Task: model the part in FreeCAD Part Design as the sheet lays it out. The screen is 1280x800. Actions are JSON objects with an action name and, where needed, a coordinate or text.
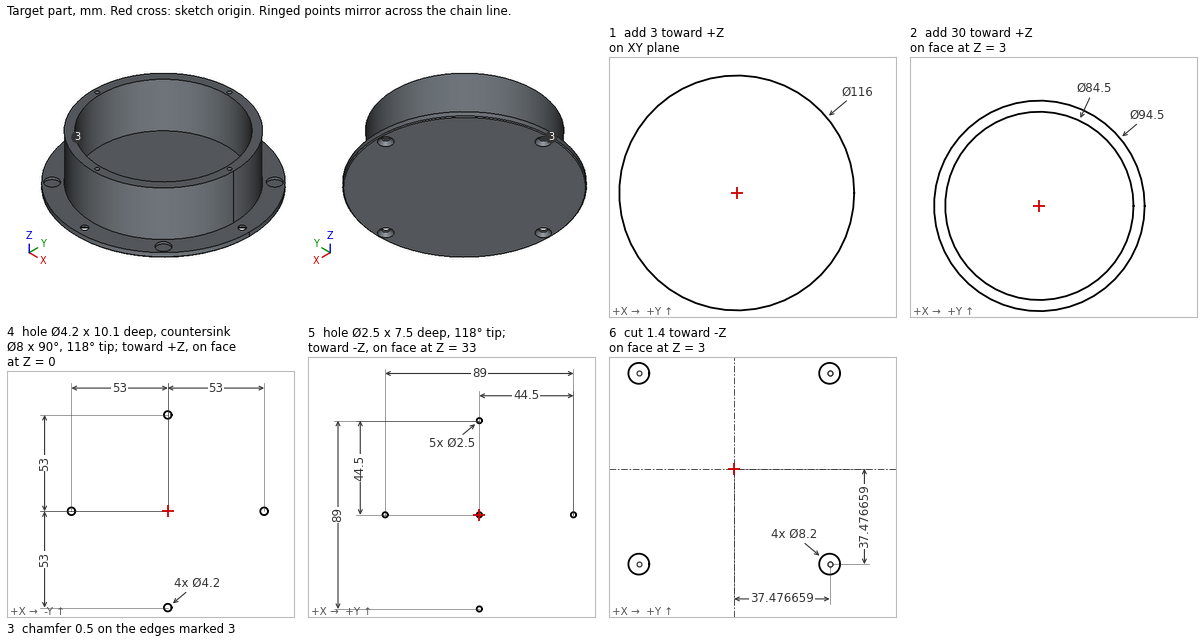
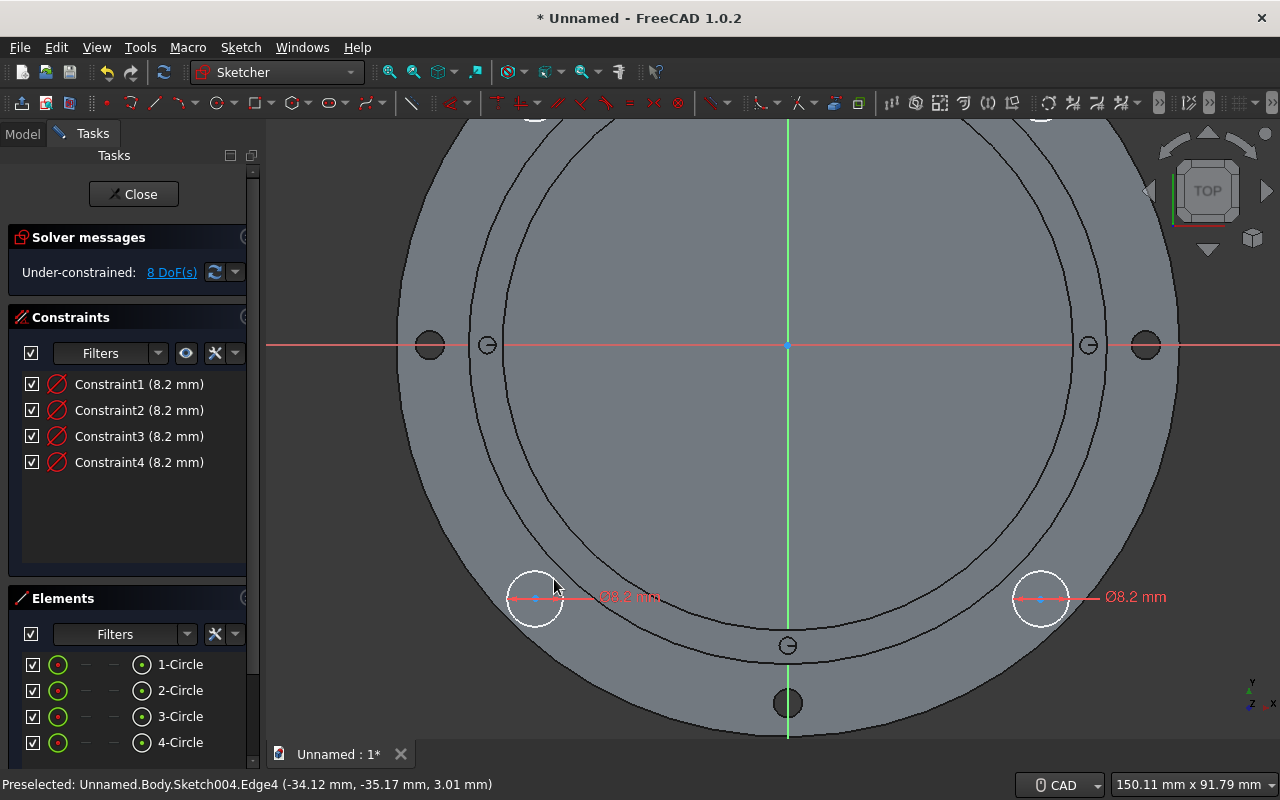
{"action": "left_click", "coordinate": [1041, 599]}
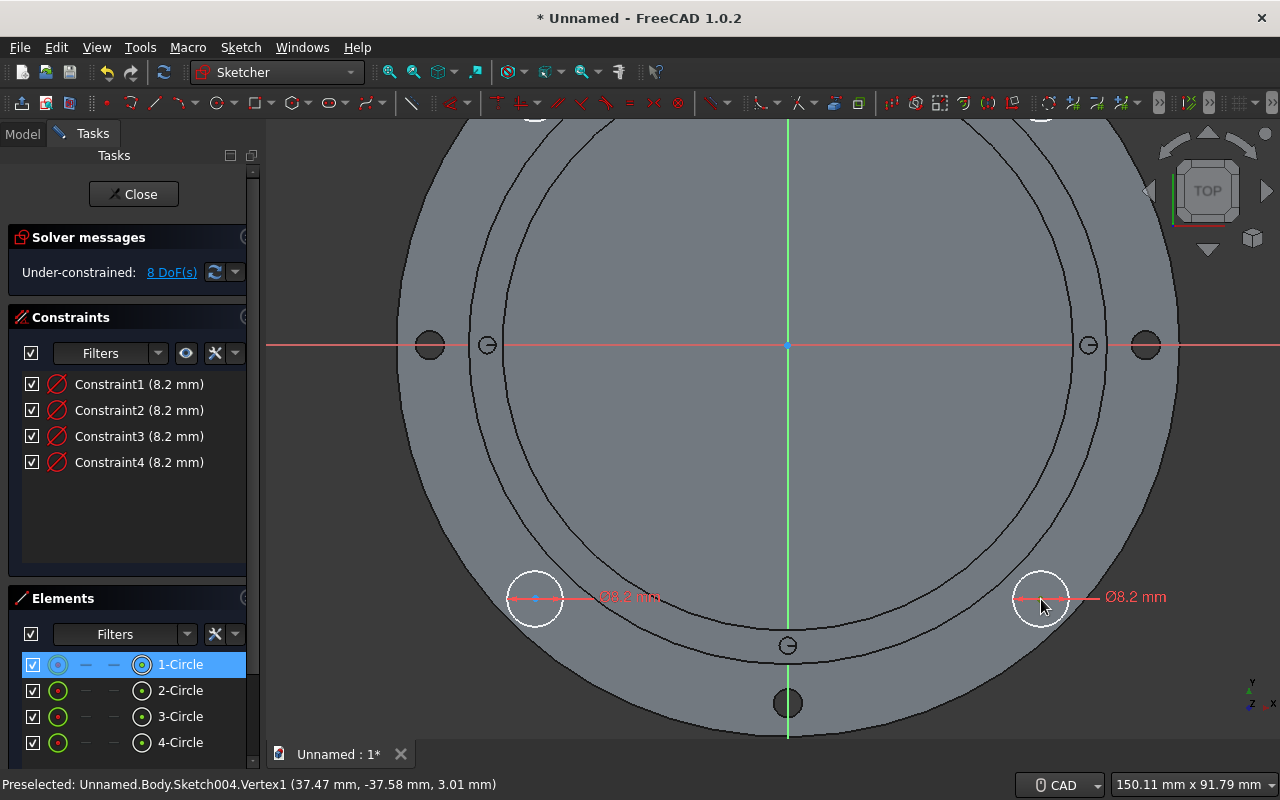
{"action": "scroll", "coordinate": [535, 599], "scroll_direction": "down", "scroll_amount": 2}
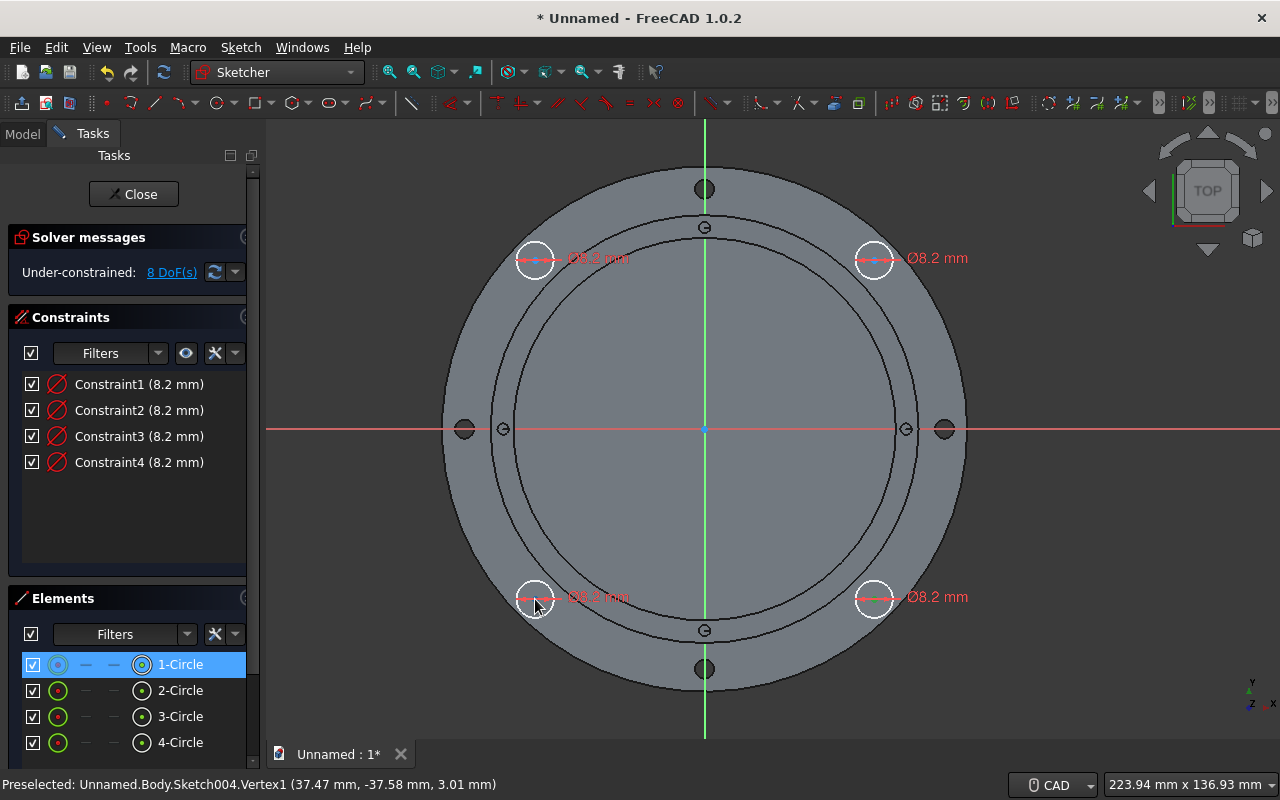
{"action": "left_click", "coordinate": [874, 260]}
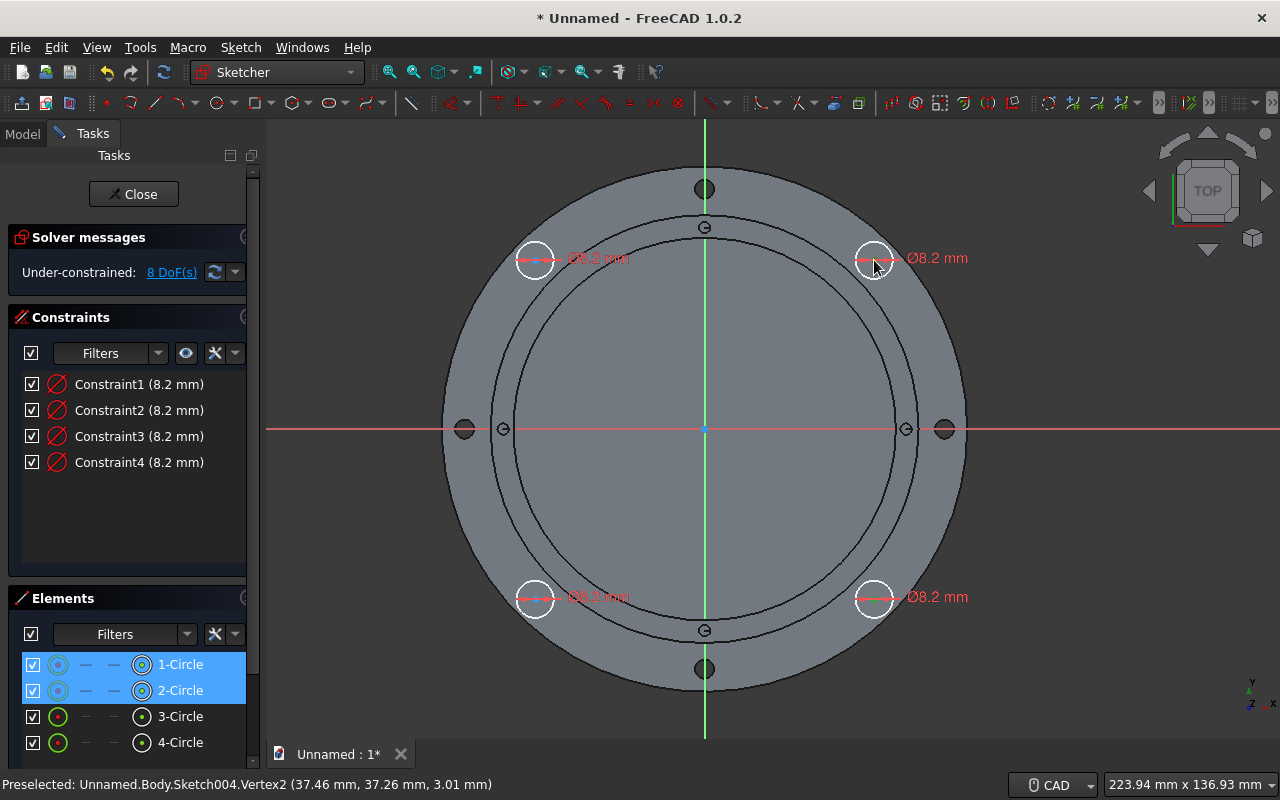
{"action": "left_click", "coordinate": [353, 429]}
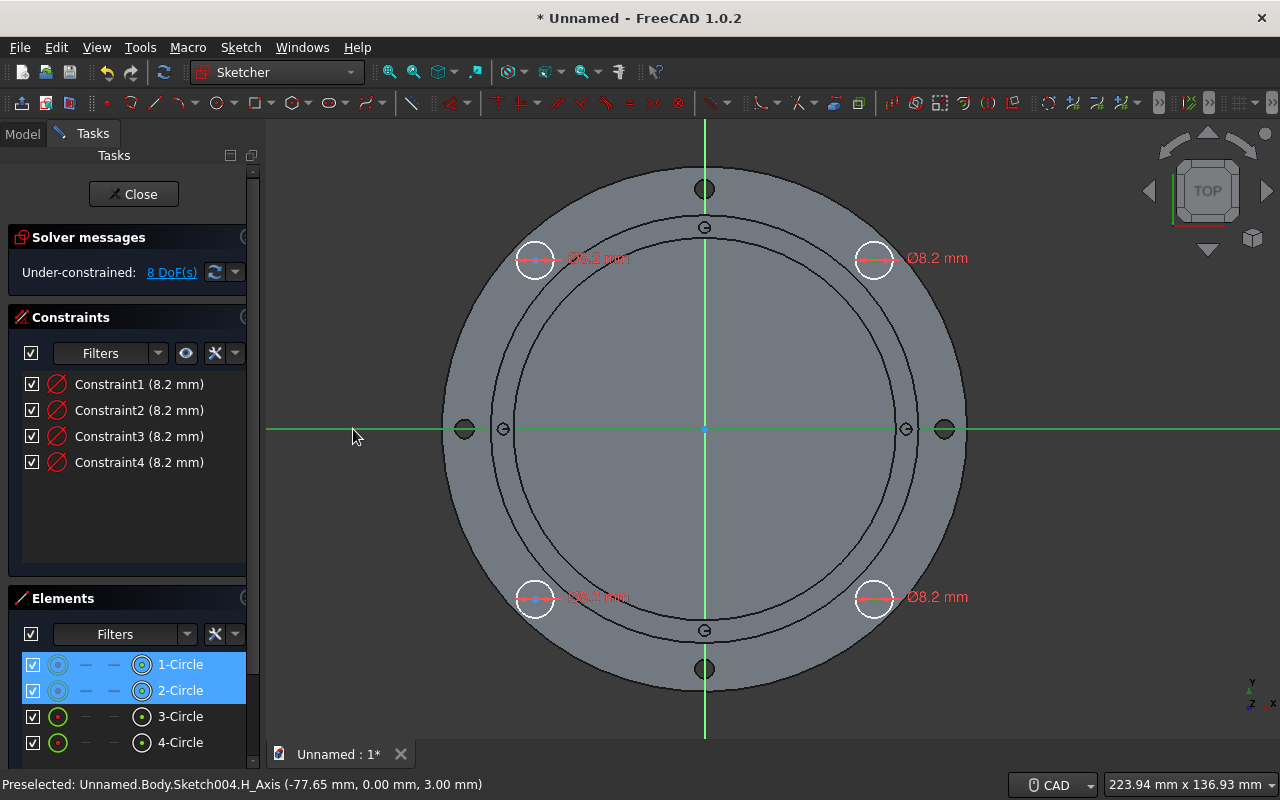
{"action": "left_click", "coordinate": [654, 104]}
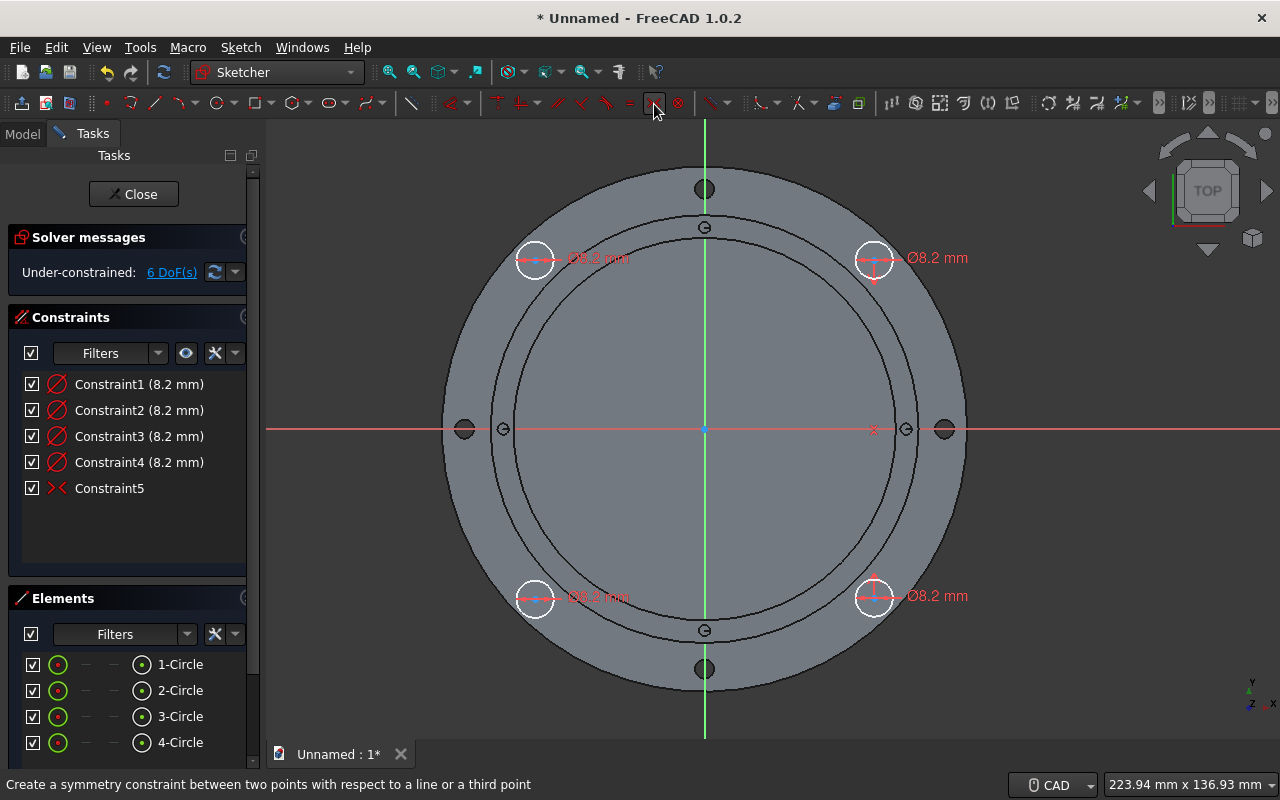
{"action": "left_click", "coordinate": [874, 260]}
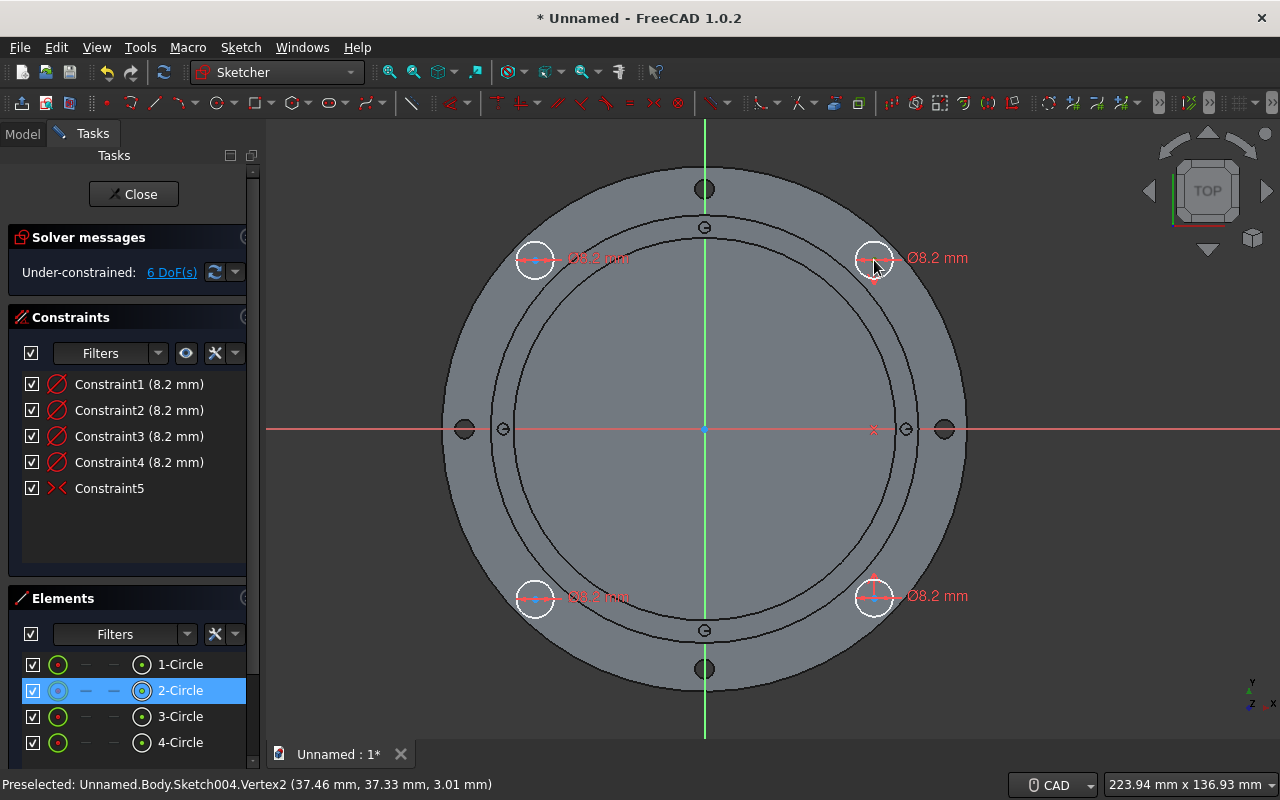
{"action": "left_click", "coordinate": [535, 260]}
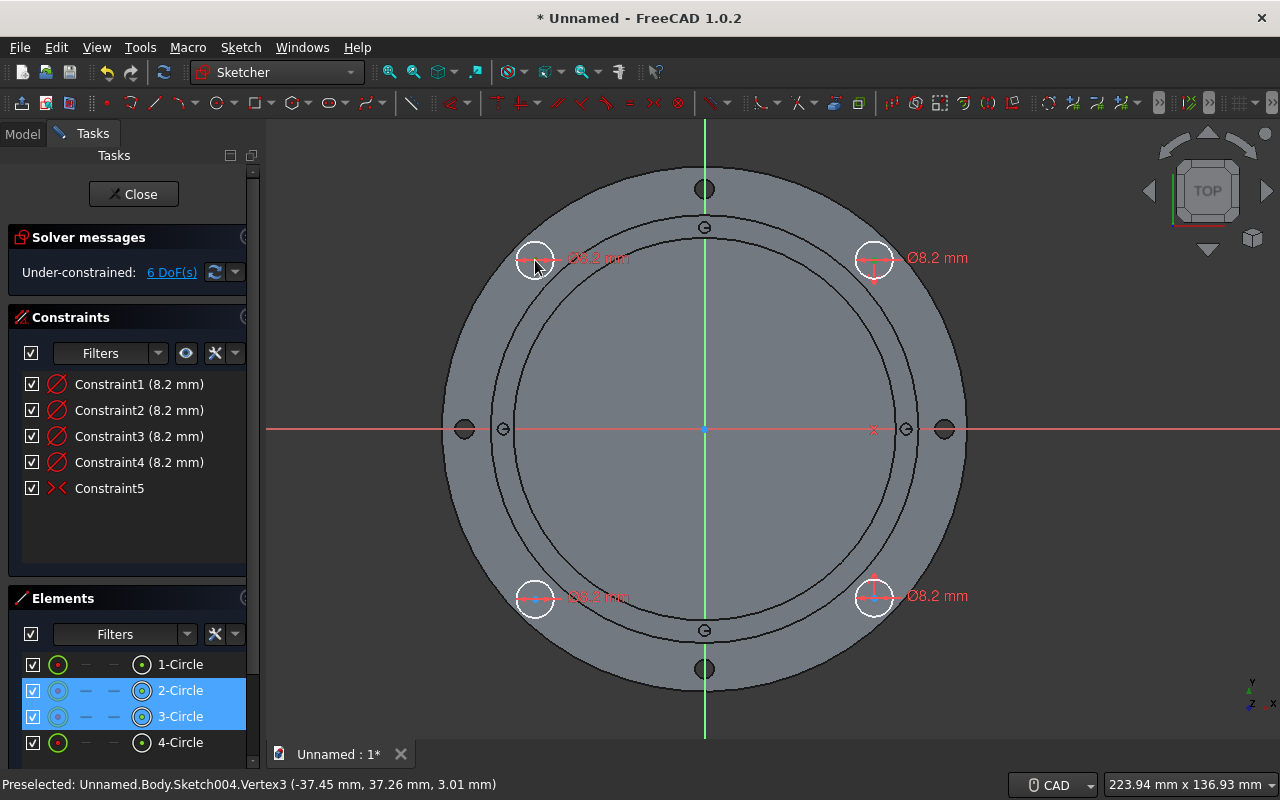
{"action": "left_click", "coordinate": [705, 671]}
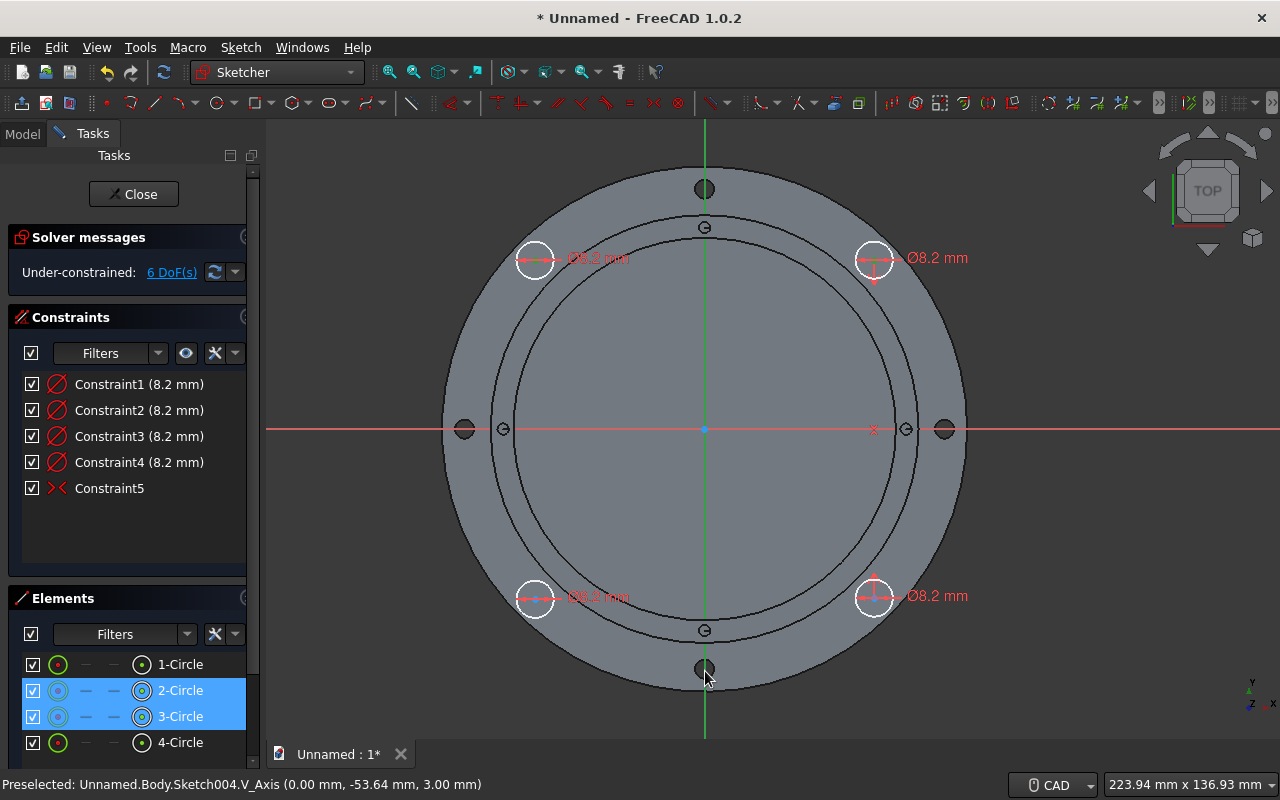
{"action": "left_click", "coordinate": [654, 104]}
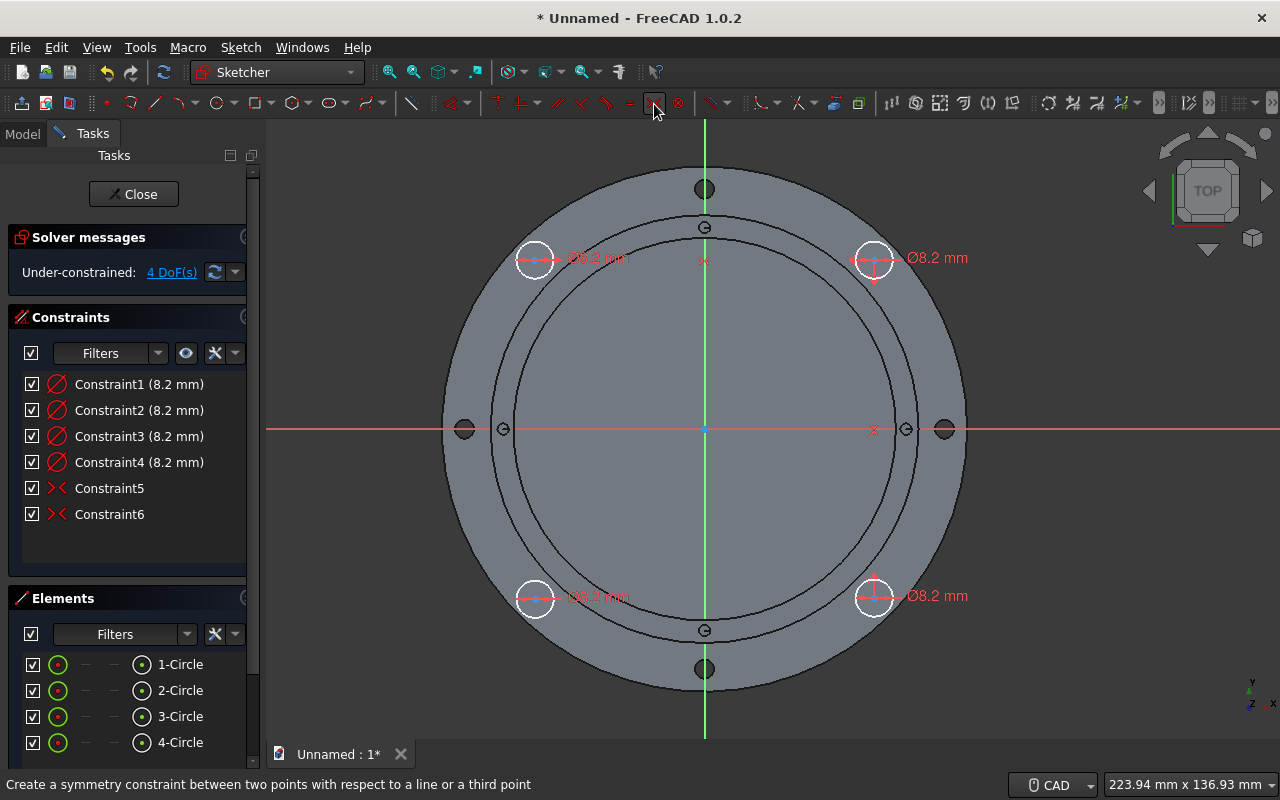
{"action": "left_click", "coordinate": [874, 598]}